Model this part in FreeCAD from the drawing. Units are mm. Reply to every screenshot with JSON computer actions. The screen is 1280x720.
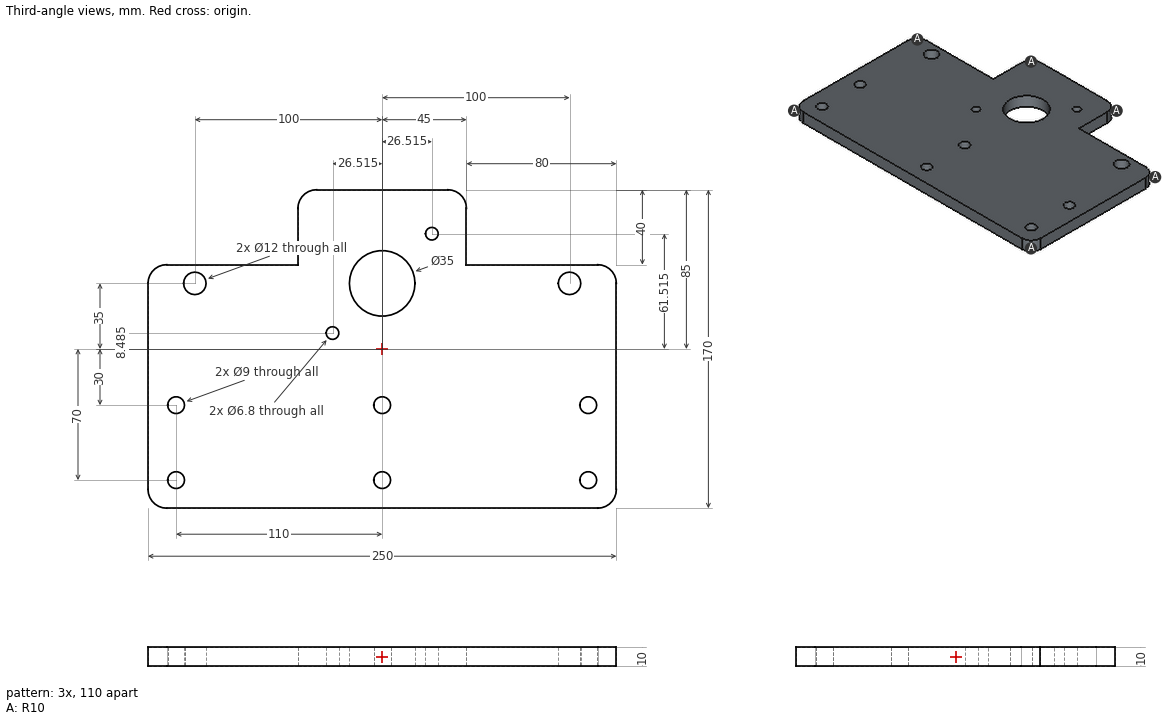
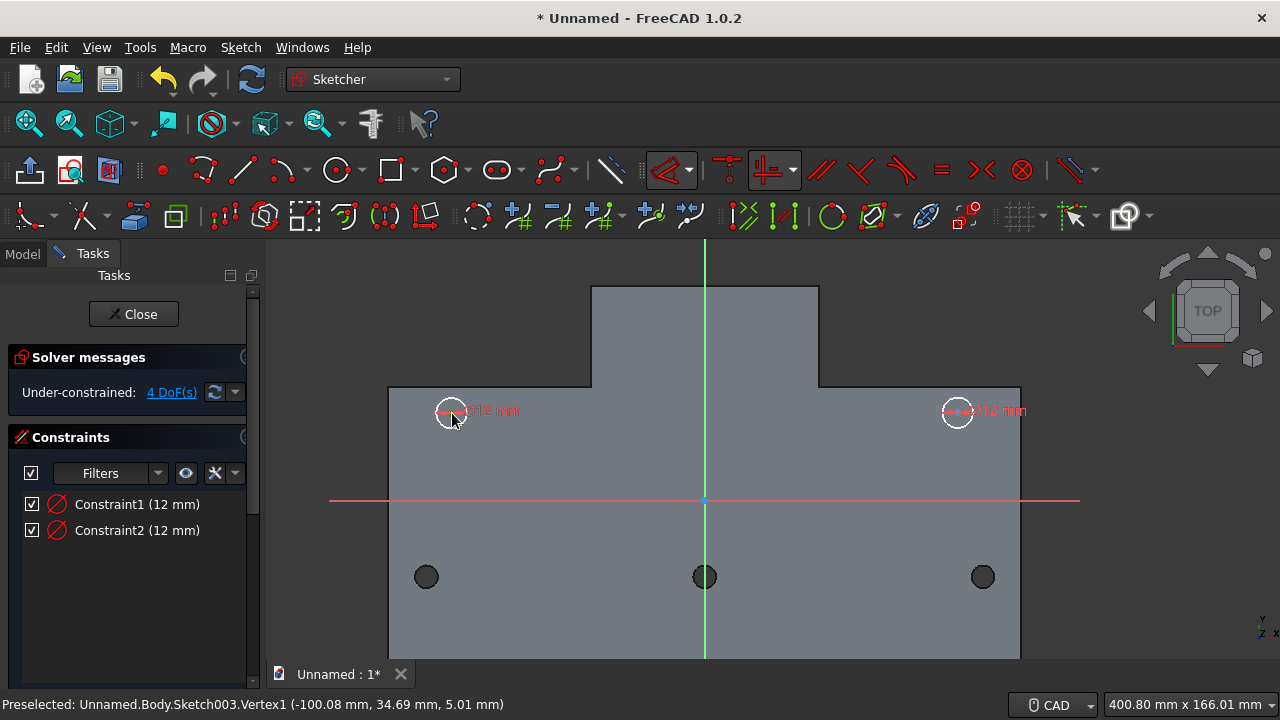
{"action": "left_click", "coordinate": [958, 413]}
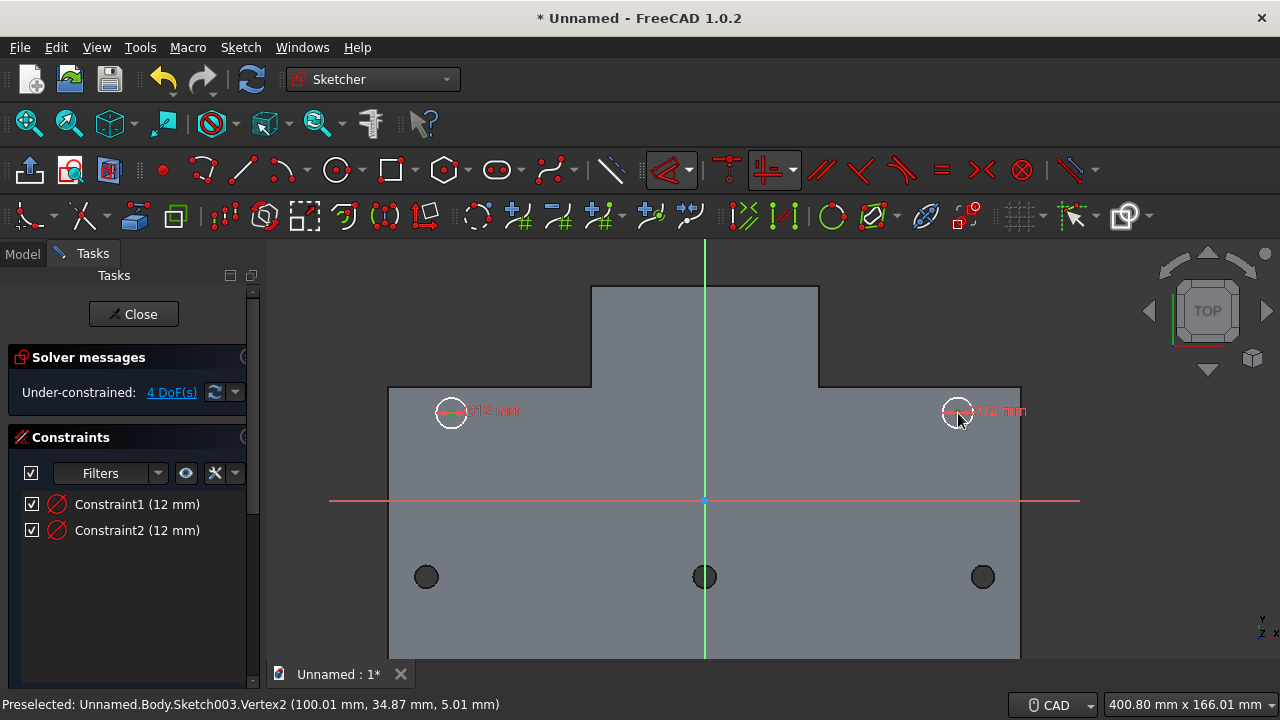
{"action": "key", "text": "h"}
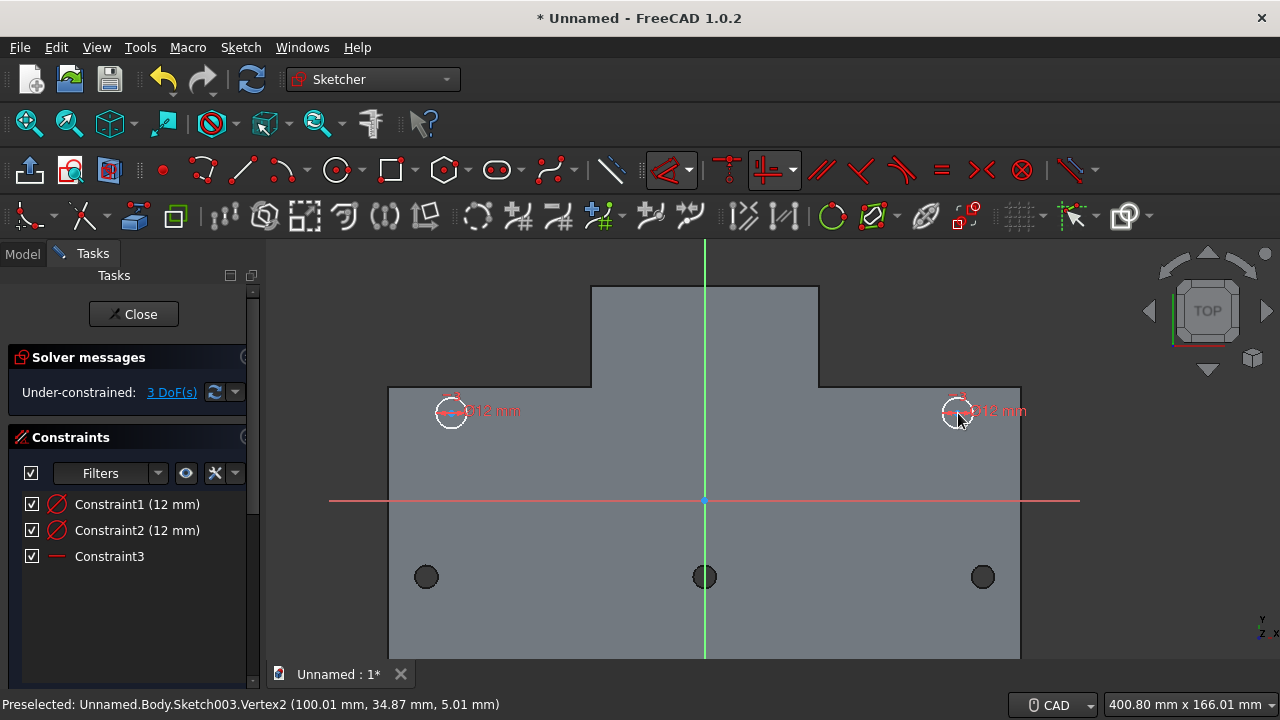
{"action": "left_click", "coordinate": [452, 413]}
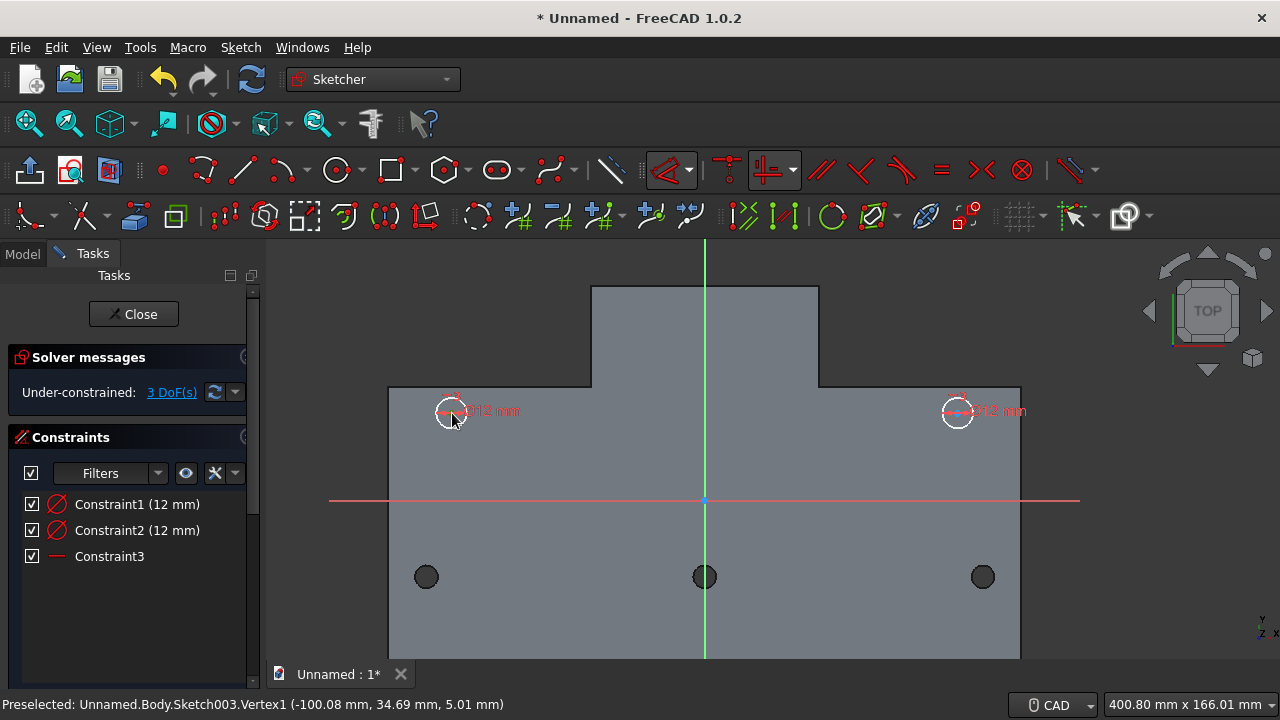
{"action": "key", "text": "i"}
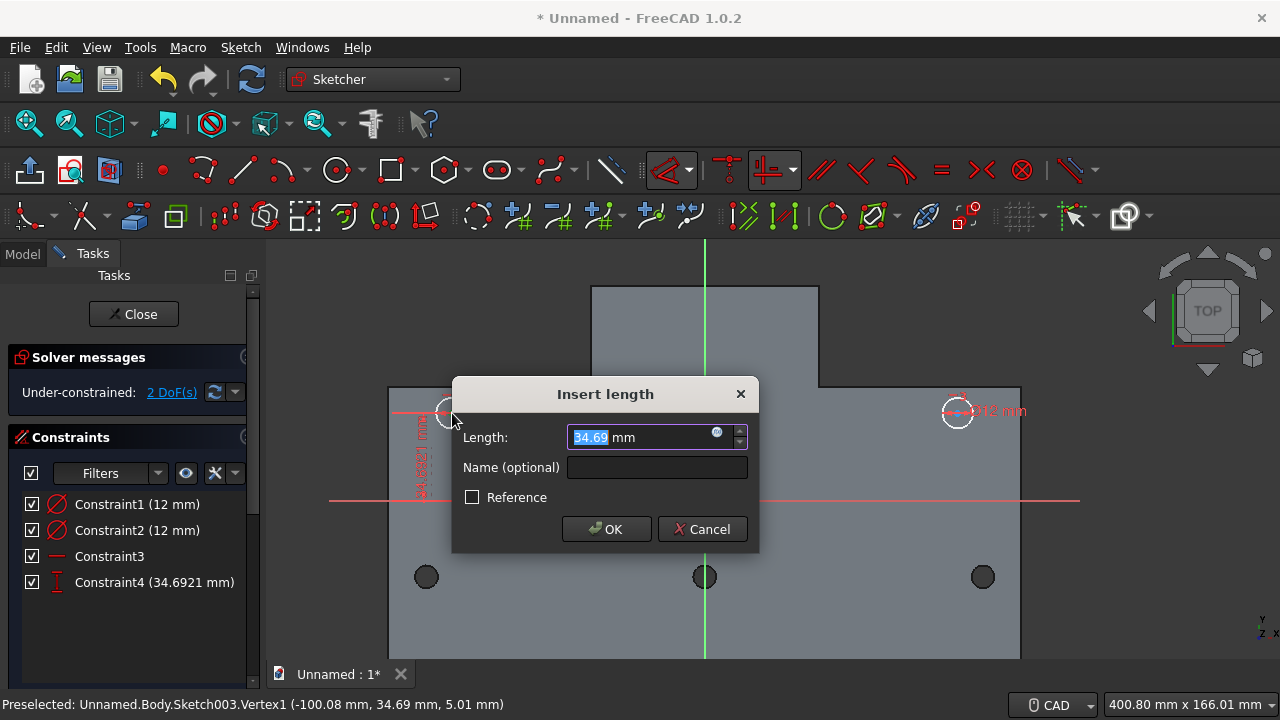
{"action": "type", "text": "35"}
{"action": "key", "text": "Return"}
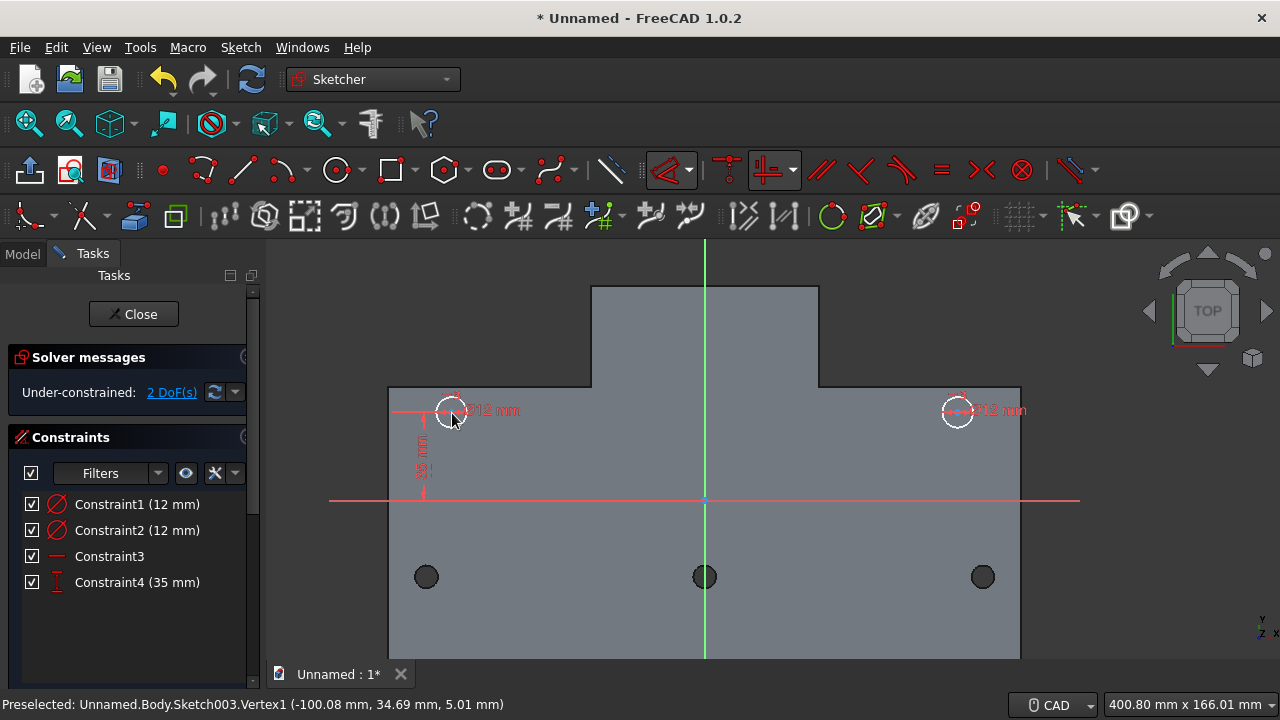
{"action": "left_click", "coordinate": [452, 412]}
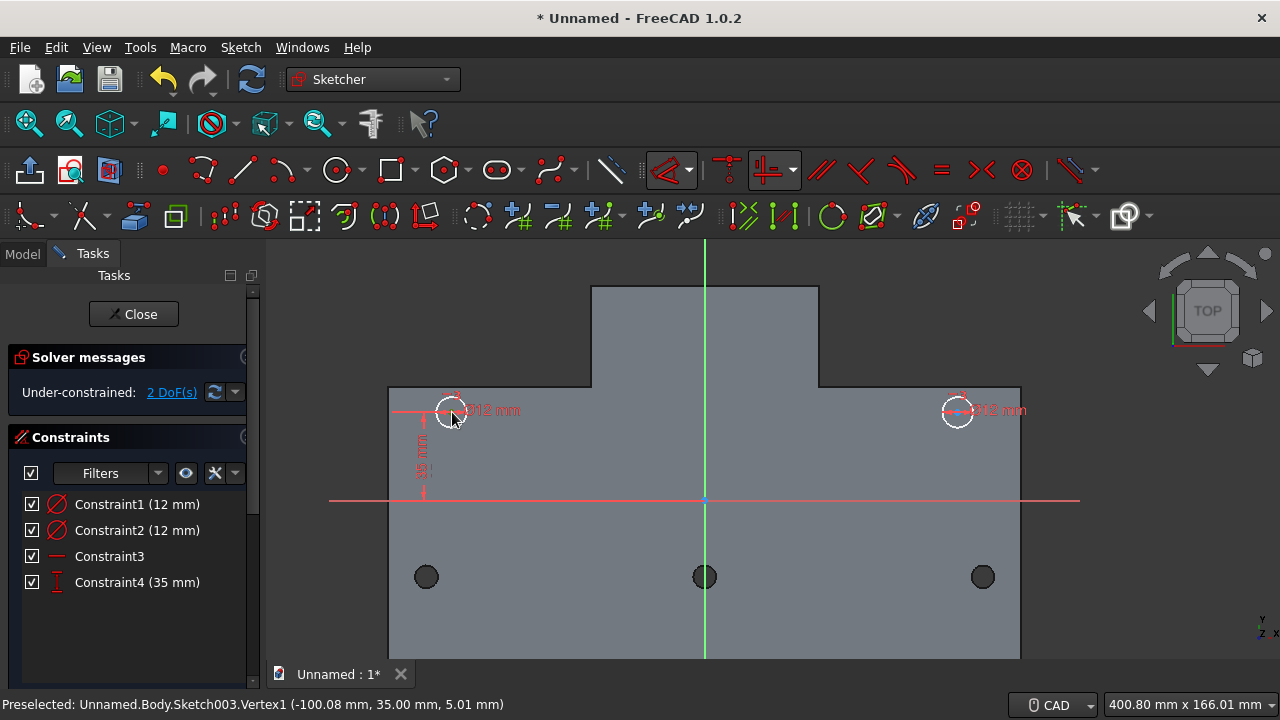
{"action": "left_click", "coordinate": [692, 170]}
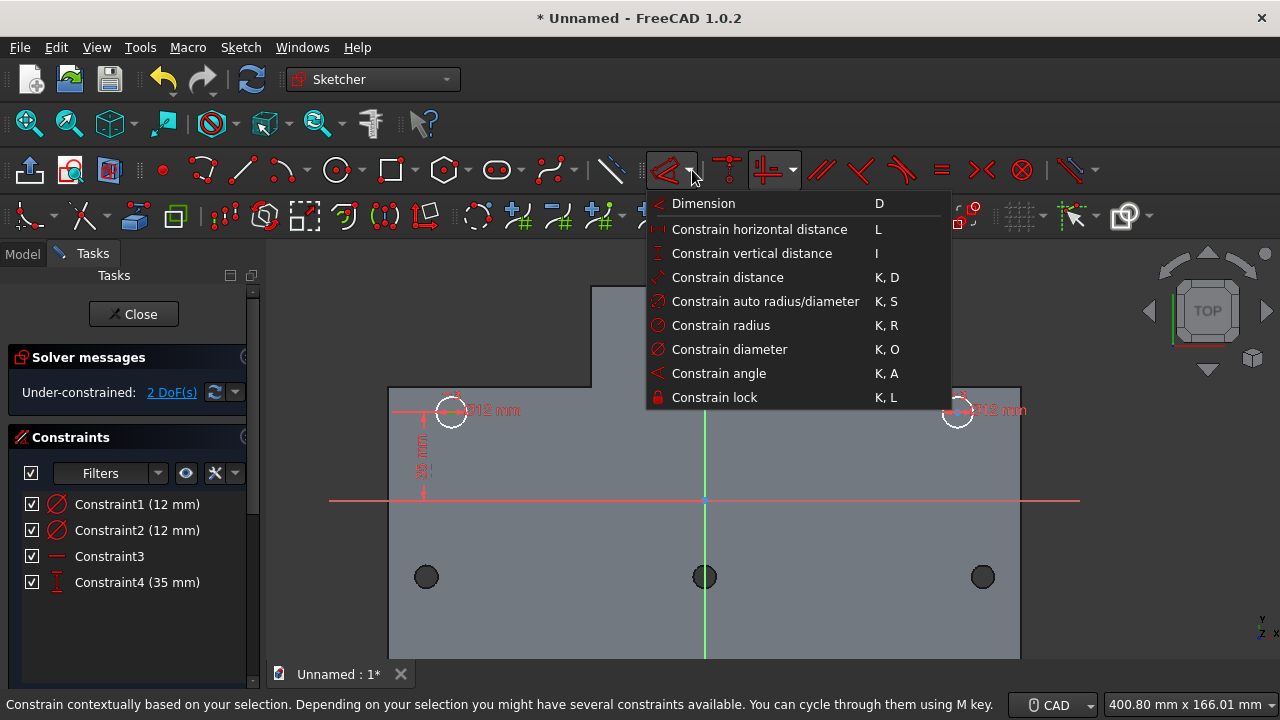
{"action": "left_click", "coordinate": [799, 229]}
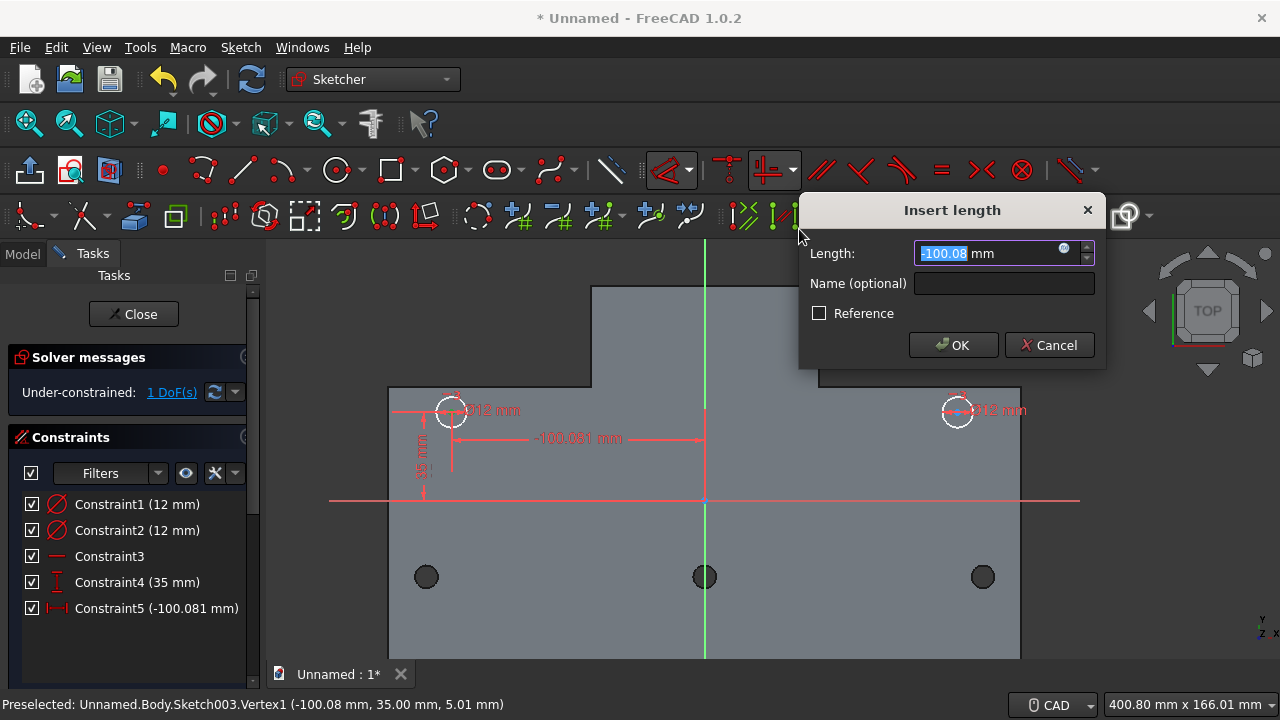
{"action": "type", "text": "-100"}
{"action": "key", "text": "Return"}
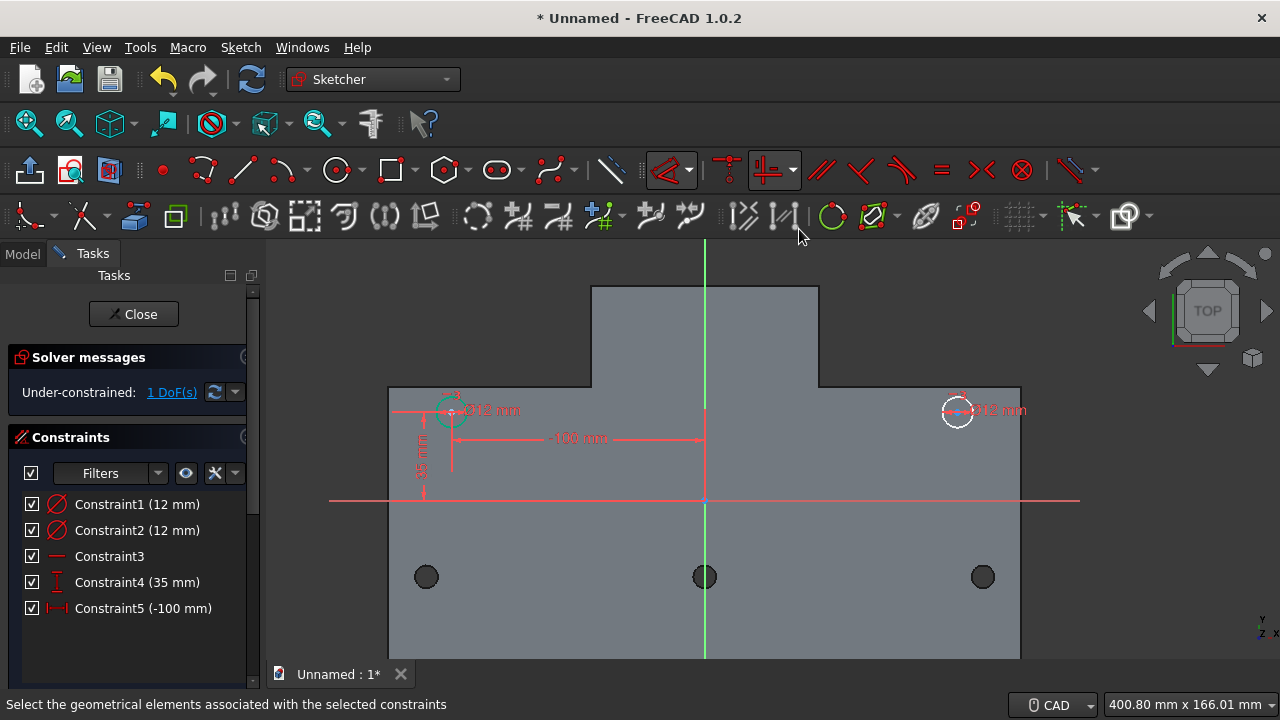
{"action": "left_click", "coordinate": [958, 412]}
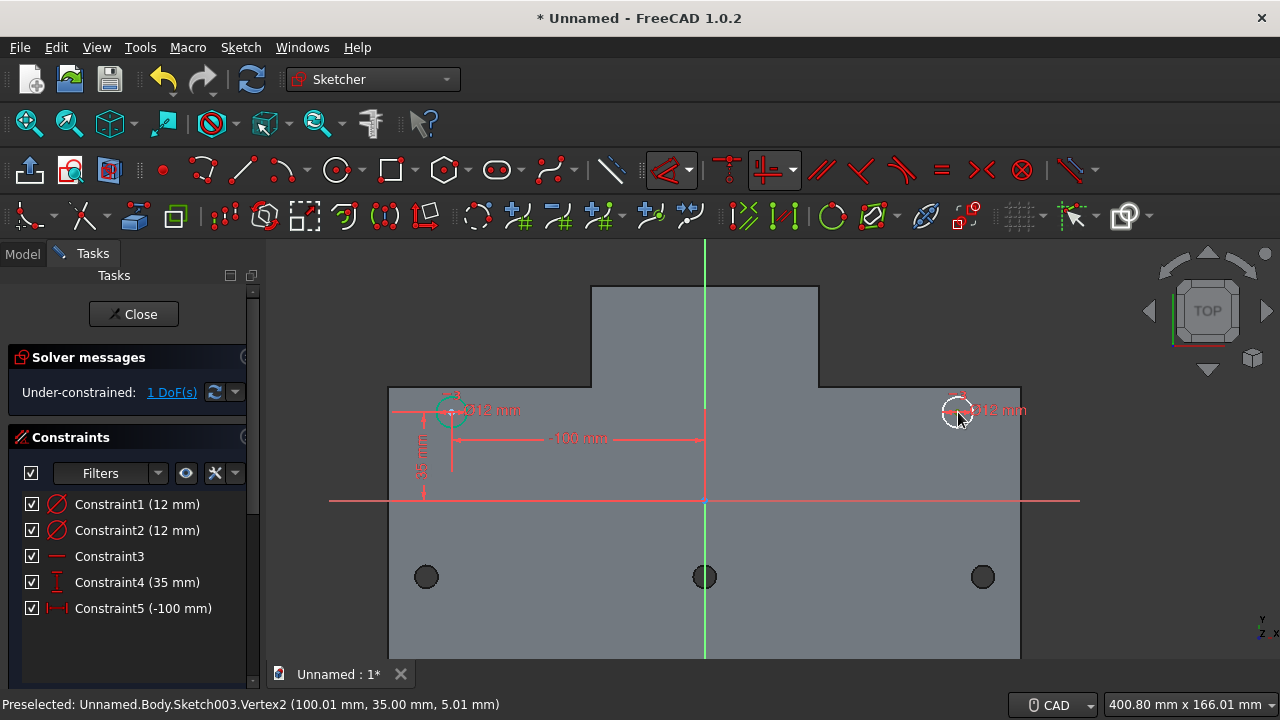
{"action": "key", "text": "l"}